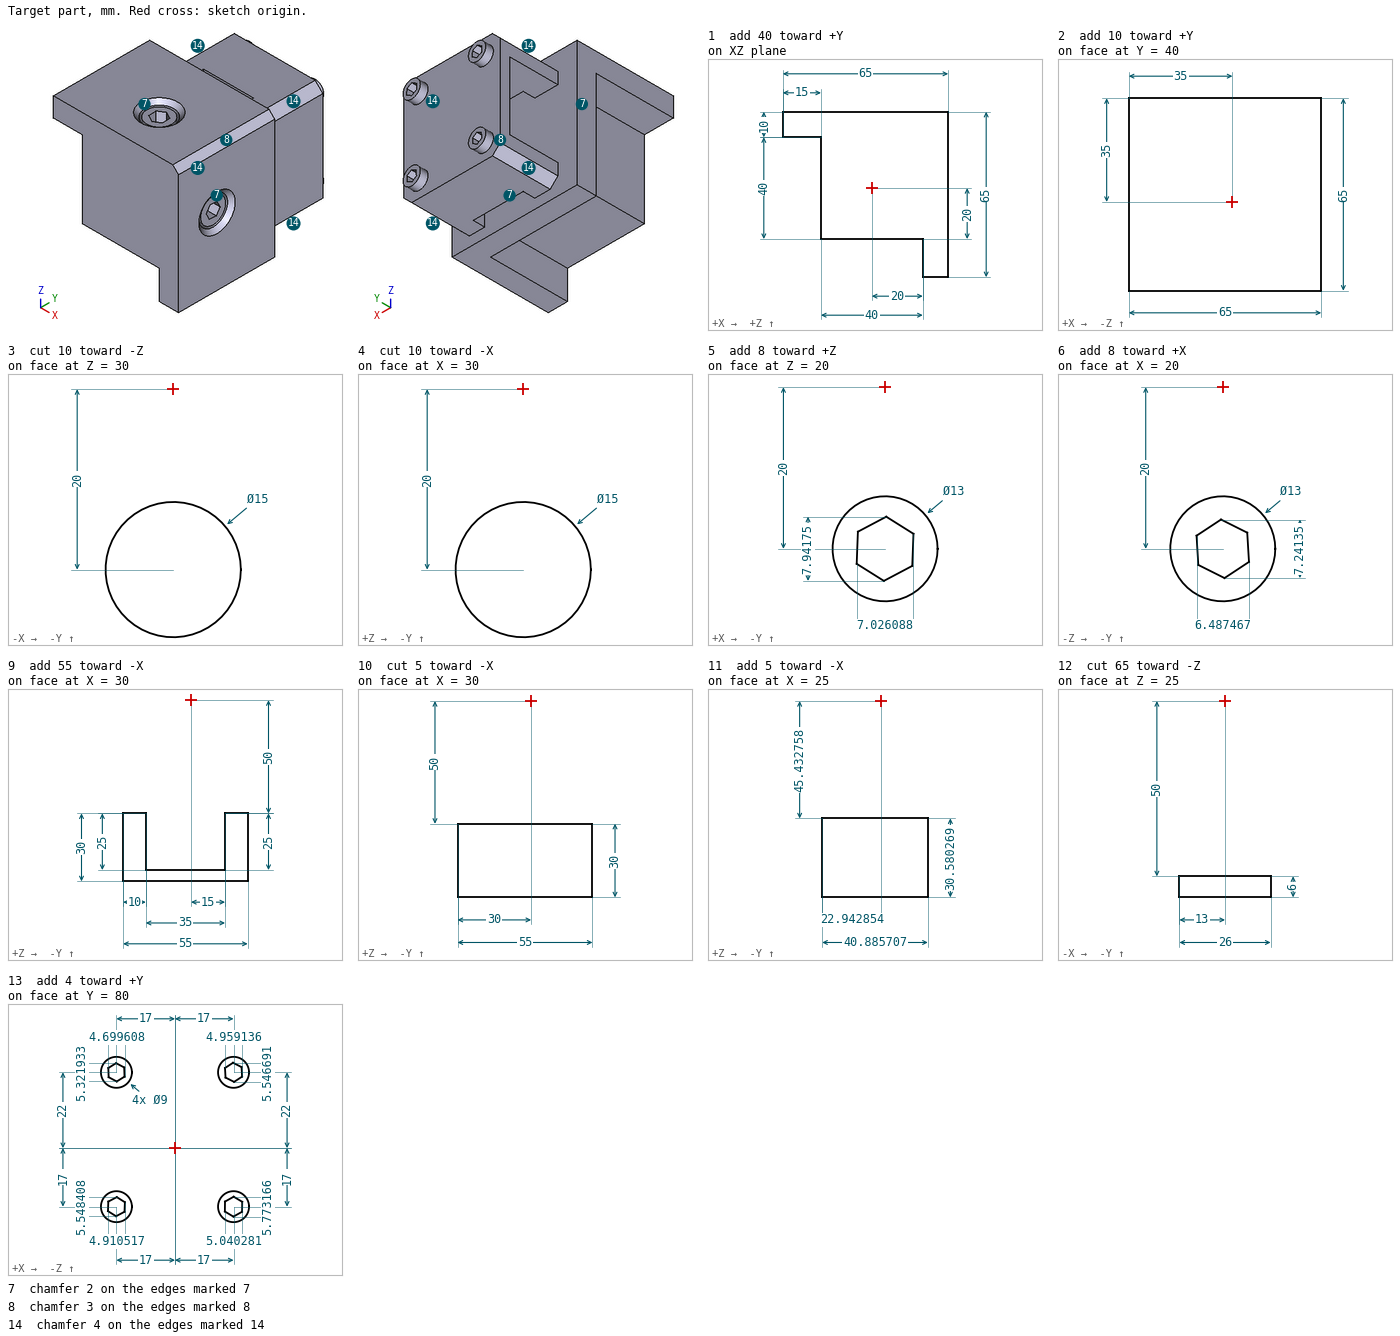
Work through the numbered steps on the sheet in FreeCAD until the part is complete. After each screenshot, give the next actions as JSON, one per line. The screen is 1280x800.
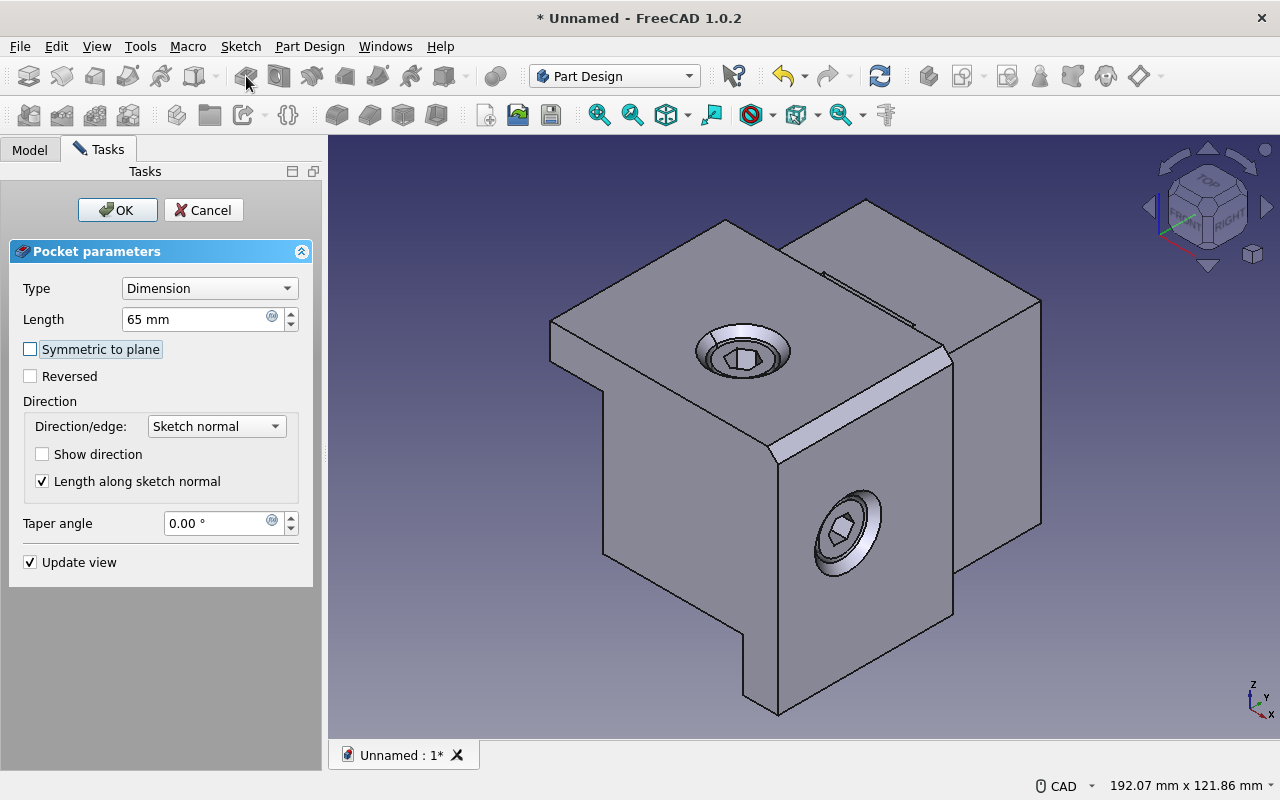
{"action": "left_click", "coordinate": [118, 210]}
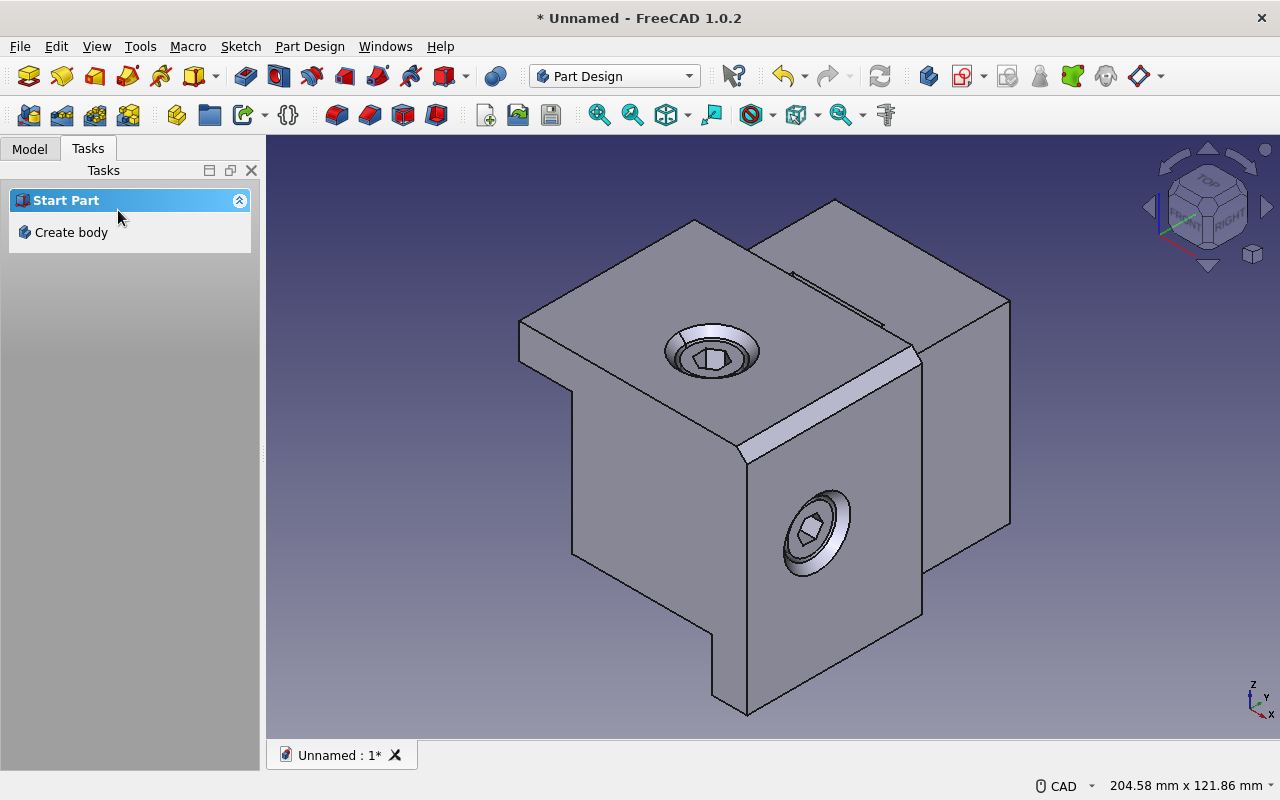
{"action": "key", "text": "4"}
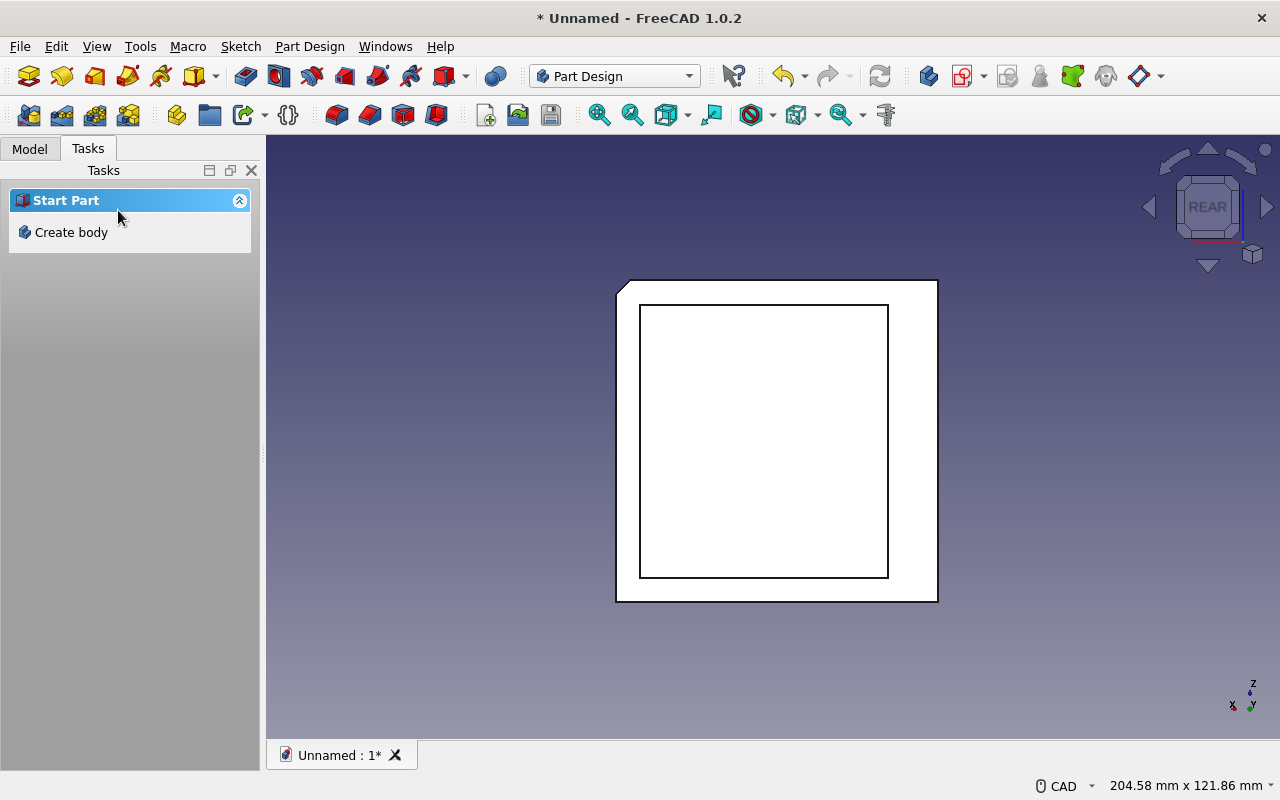
{"action": "left_click", "coordinate": [764, 440]}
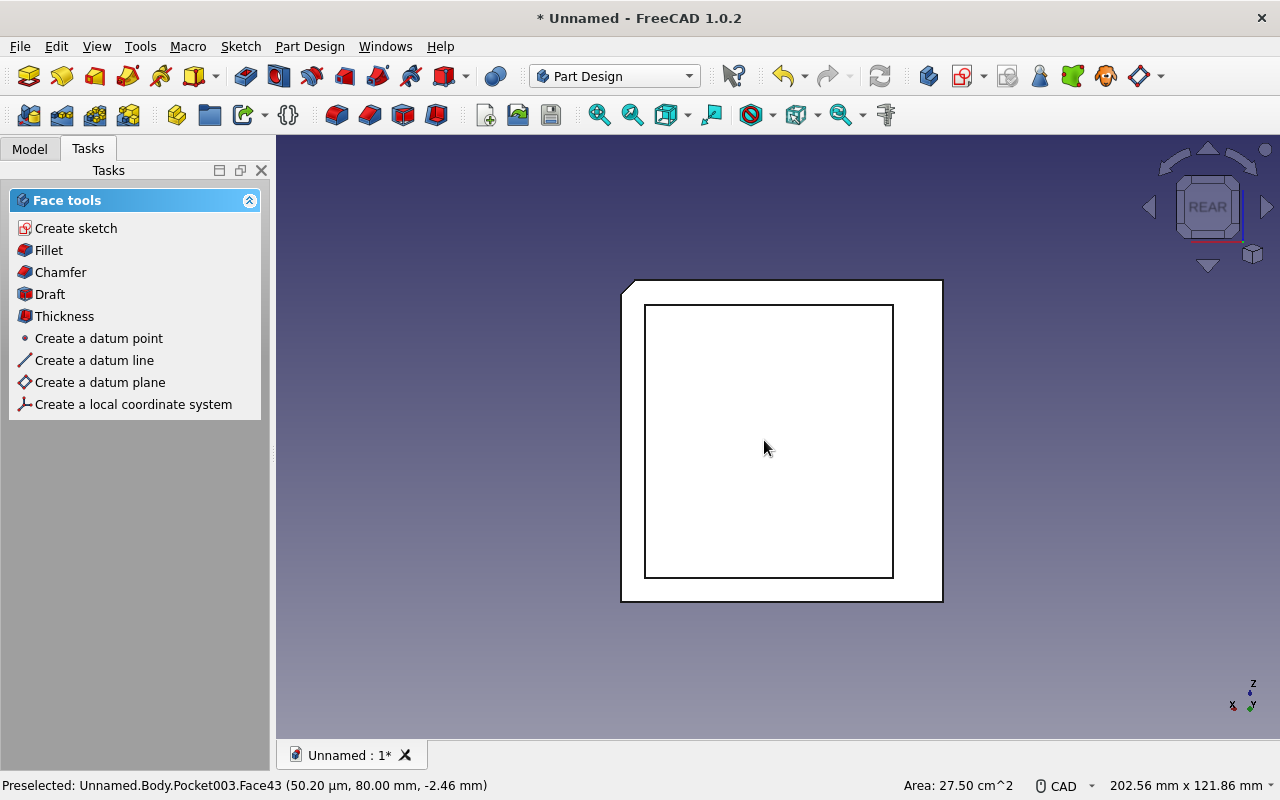
{"action": "left_click", "coordinate": [962, 76]}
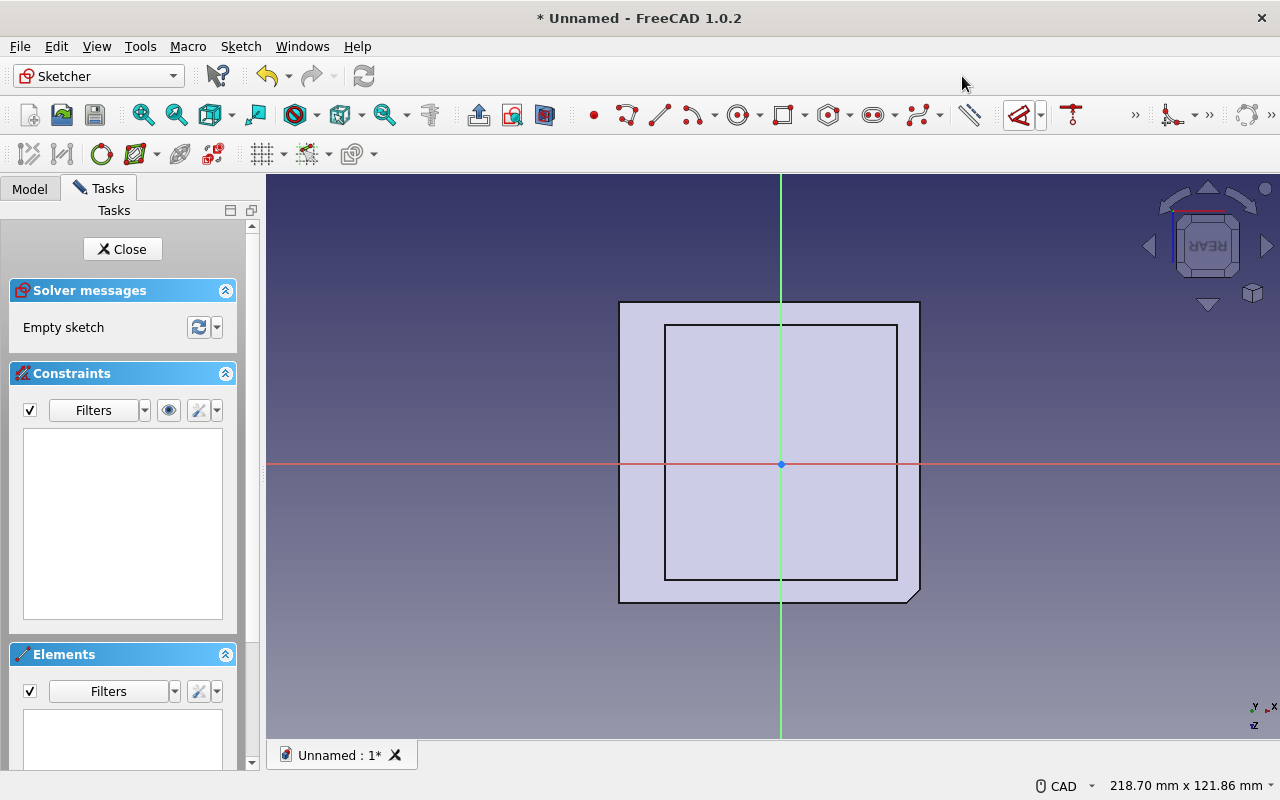
{"action": "scroll", "coordinate": [937, 445], "scroll_direction": "up", "scroll_amount": 2}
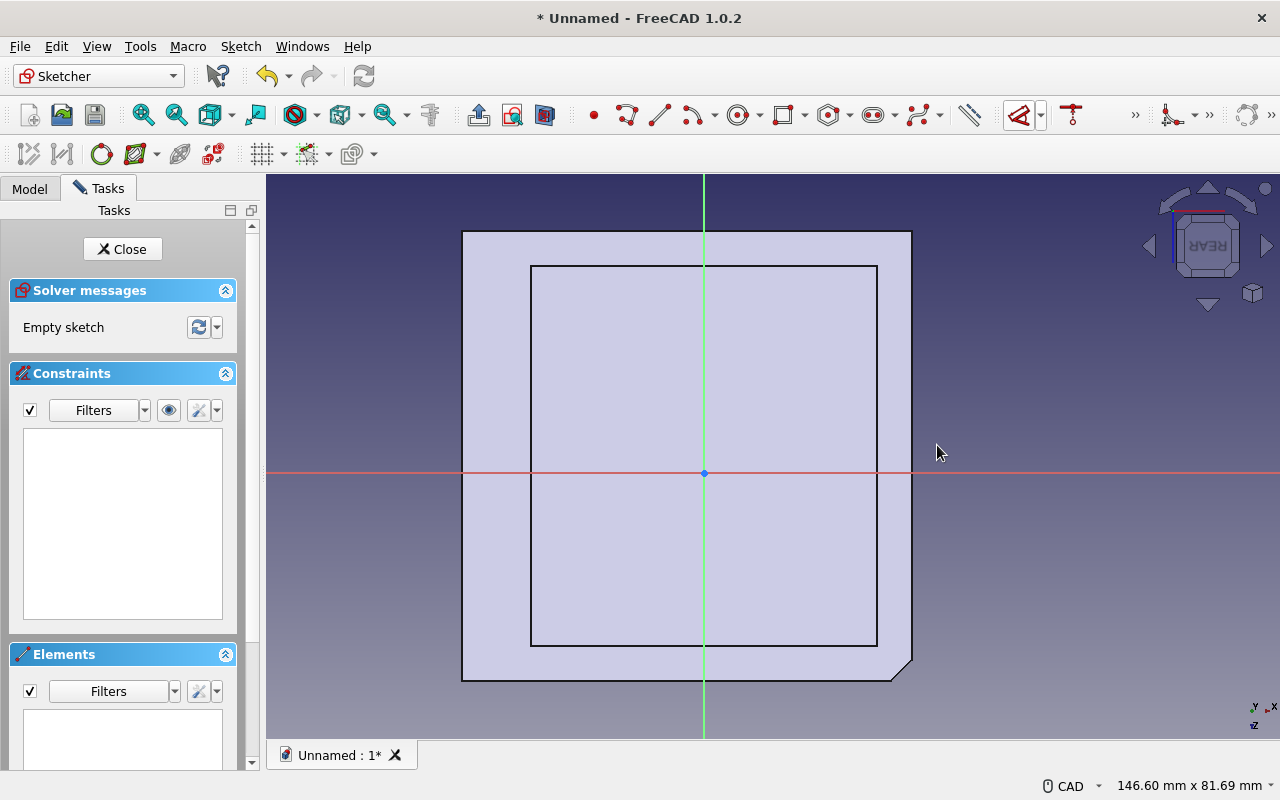
{"action": "left_click", "coordinate": [828, 116]}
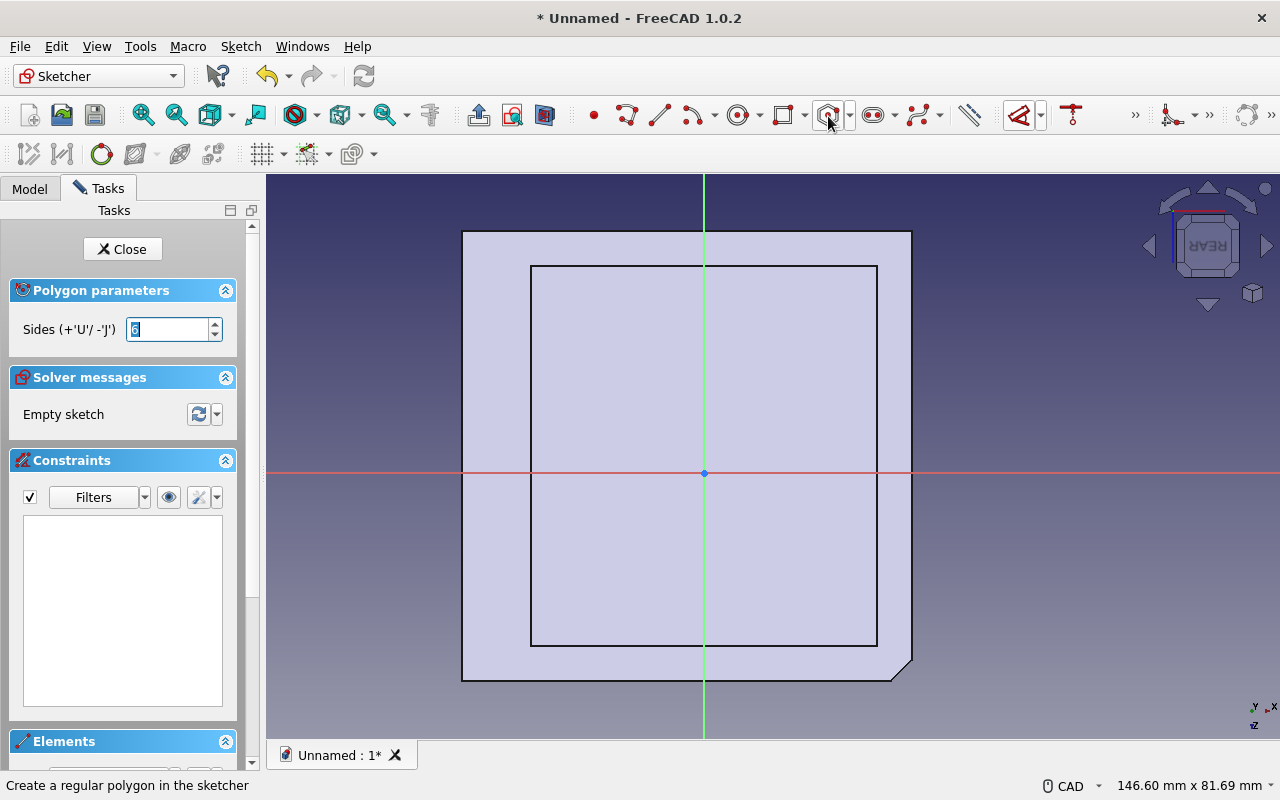
{"action": "scroll", "coordinate": [587, 321], "scroll_direction": "up", "scroll_amount": 3}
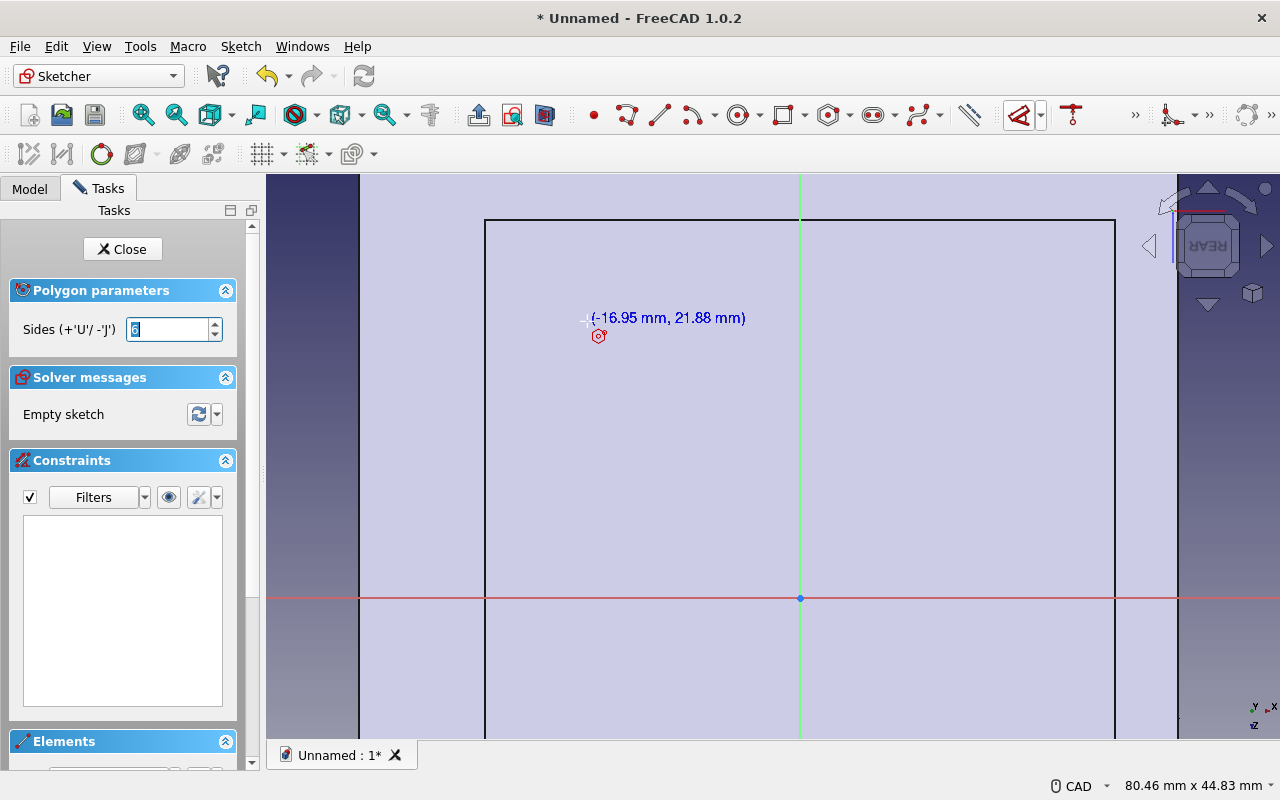
{"action": "left_click", "coordinate": [586, 321]}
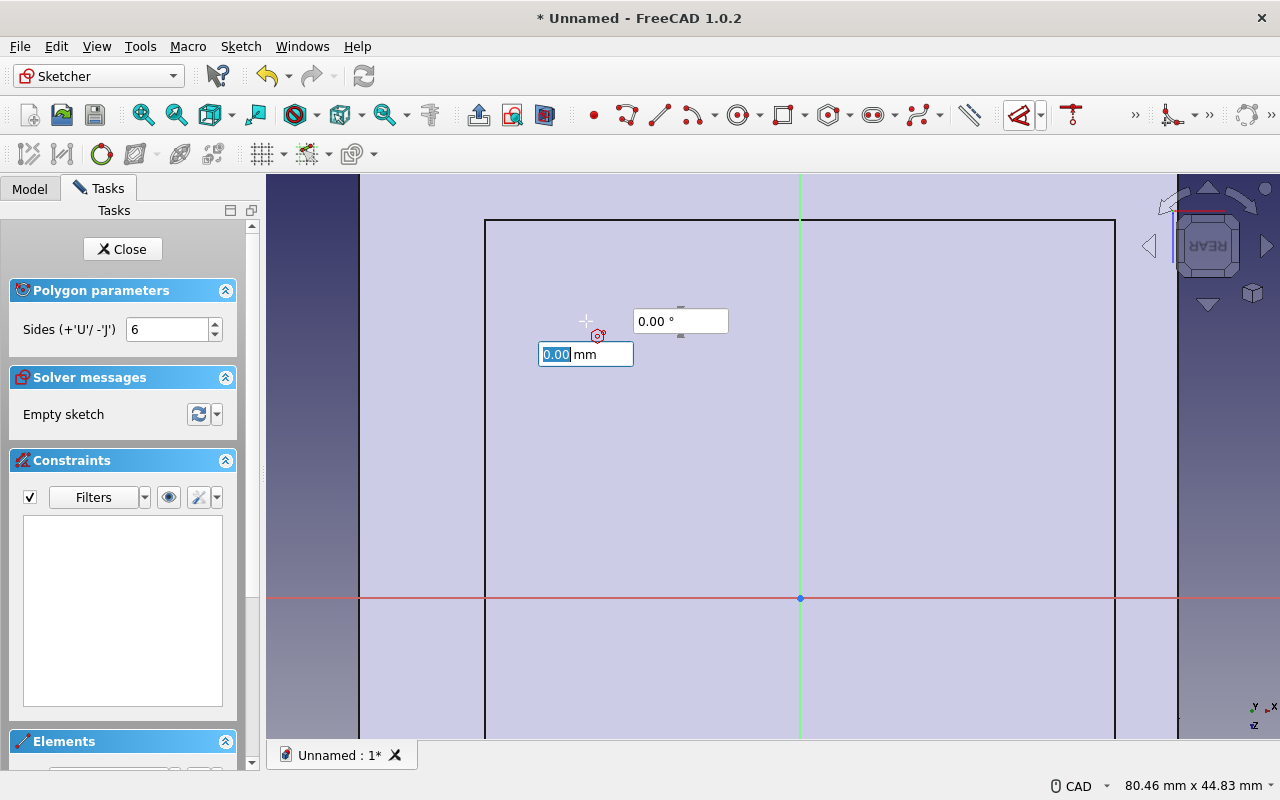
{"action": "left_click", "coordinate": [556, 305]}
{"action": "right_click", "coordinate": [556, 305]}